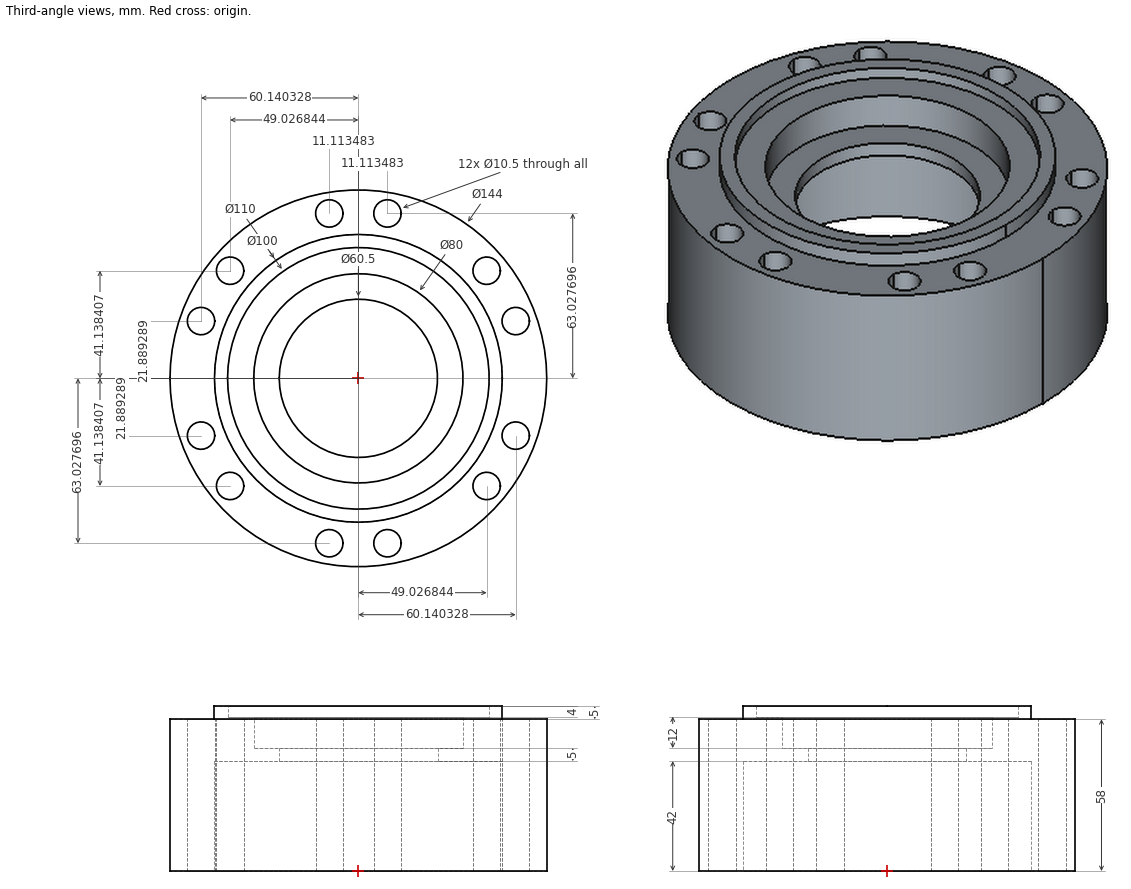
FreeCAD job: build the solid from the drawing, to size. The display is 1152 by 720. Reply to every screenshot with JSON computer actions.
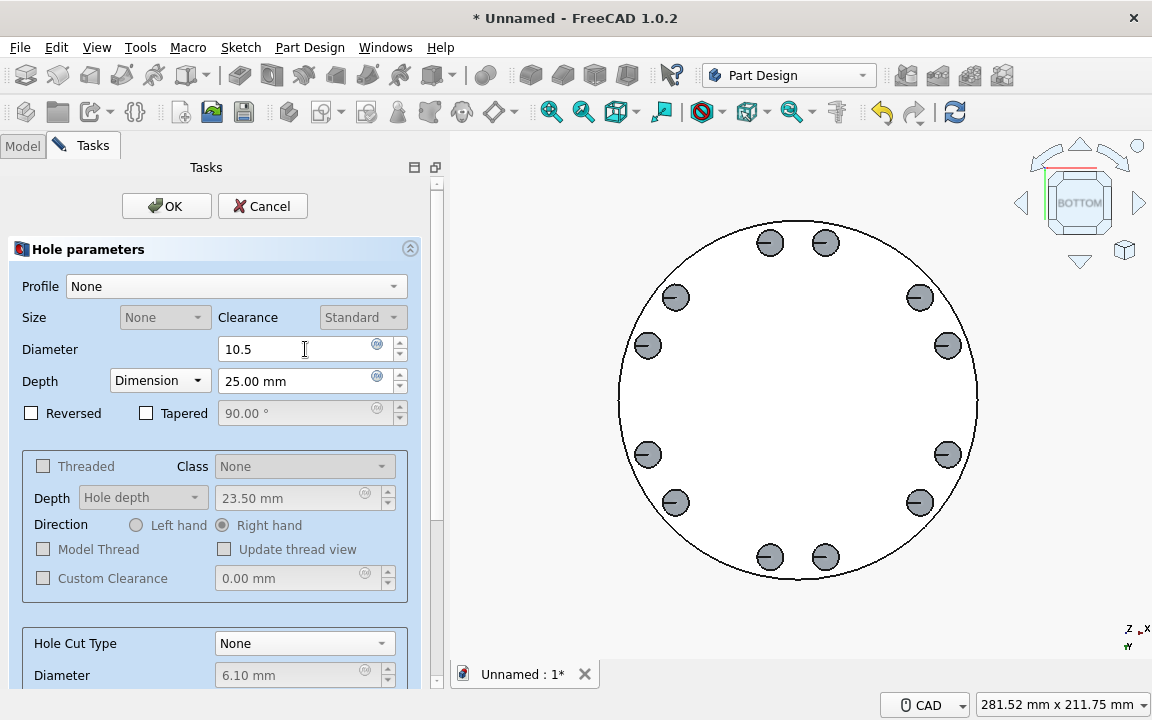
{"action": "left_click", "coordinate": [161, 380]}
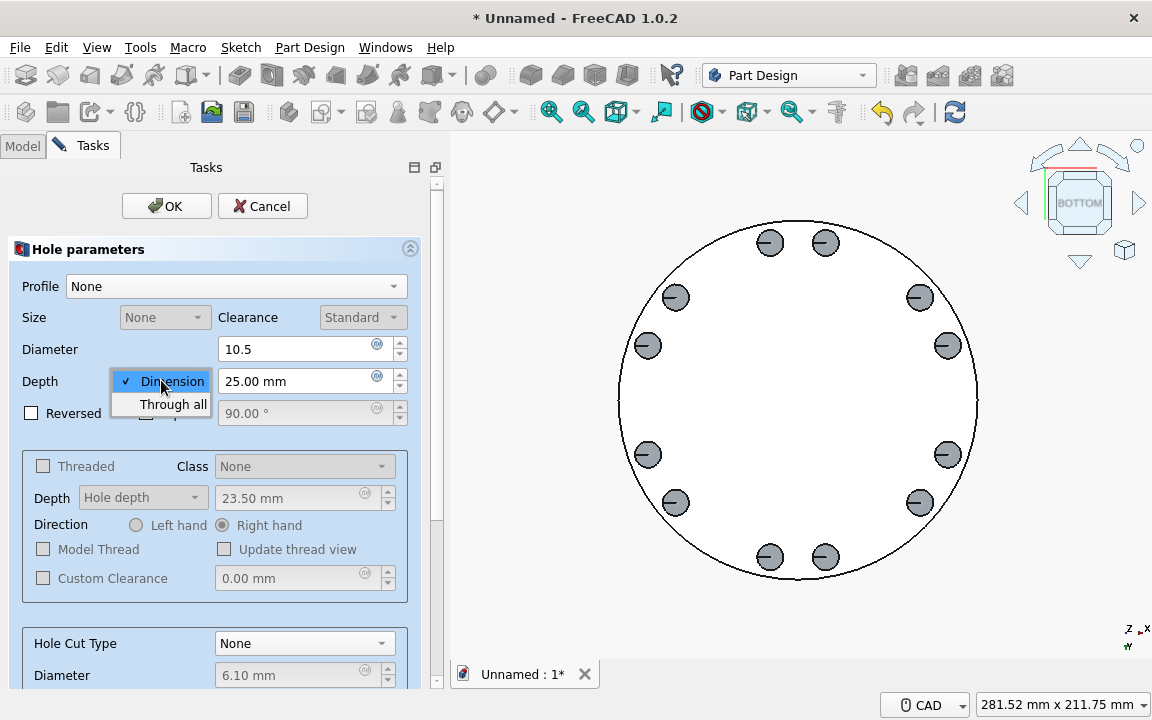
{"action": "left_click", "coordinate": [160, 404]}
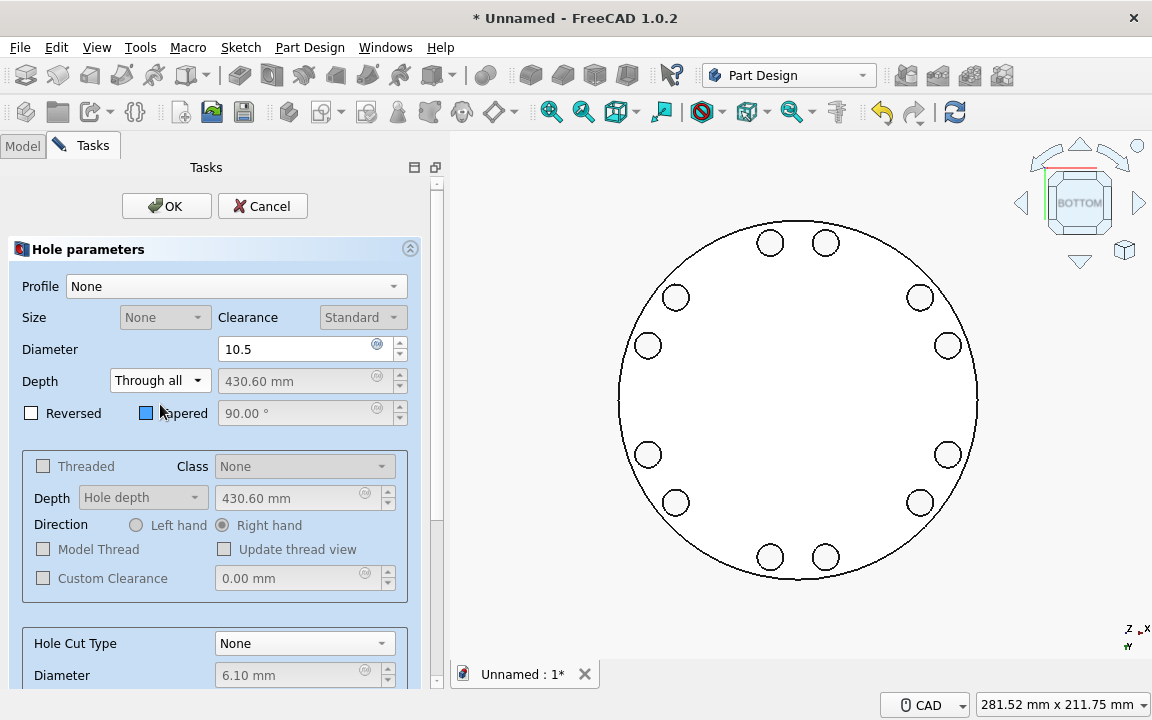
{"action": "left_click", "coordinate": [167, 206]}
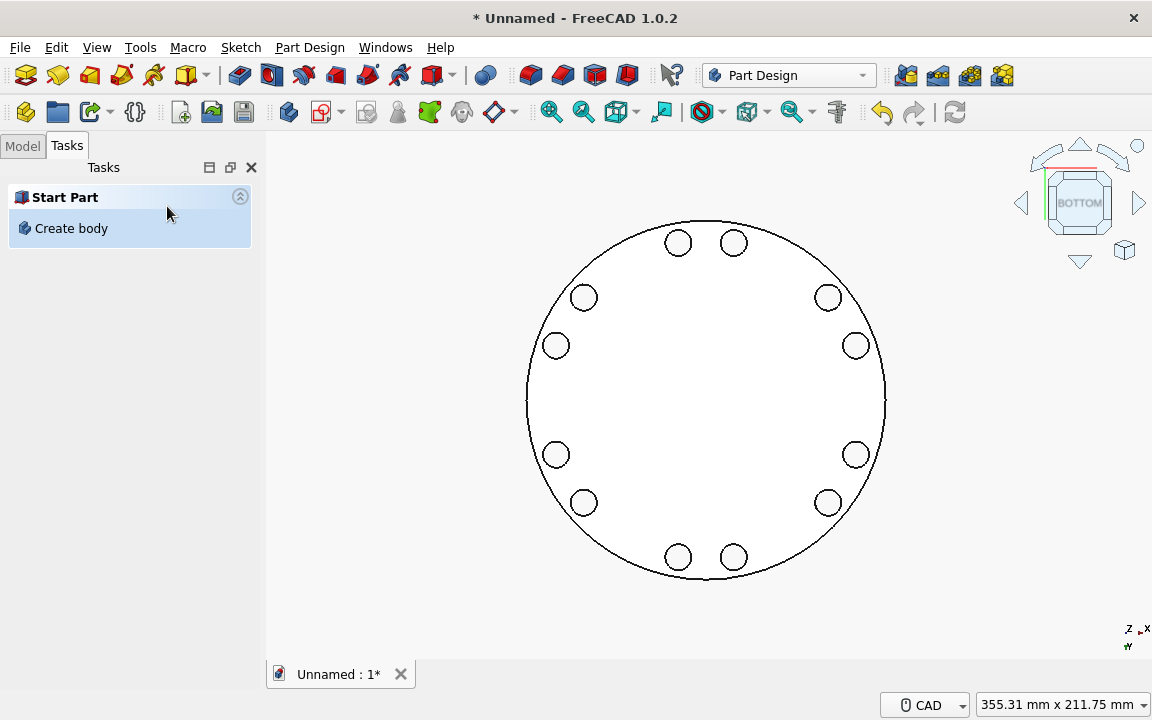
{"action": "left_click", "coordinate": [706, 399]}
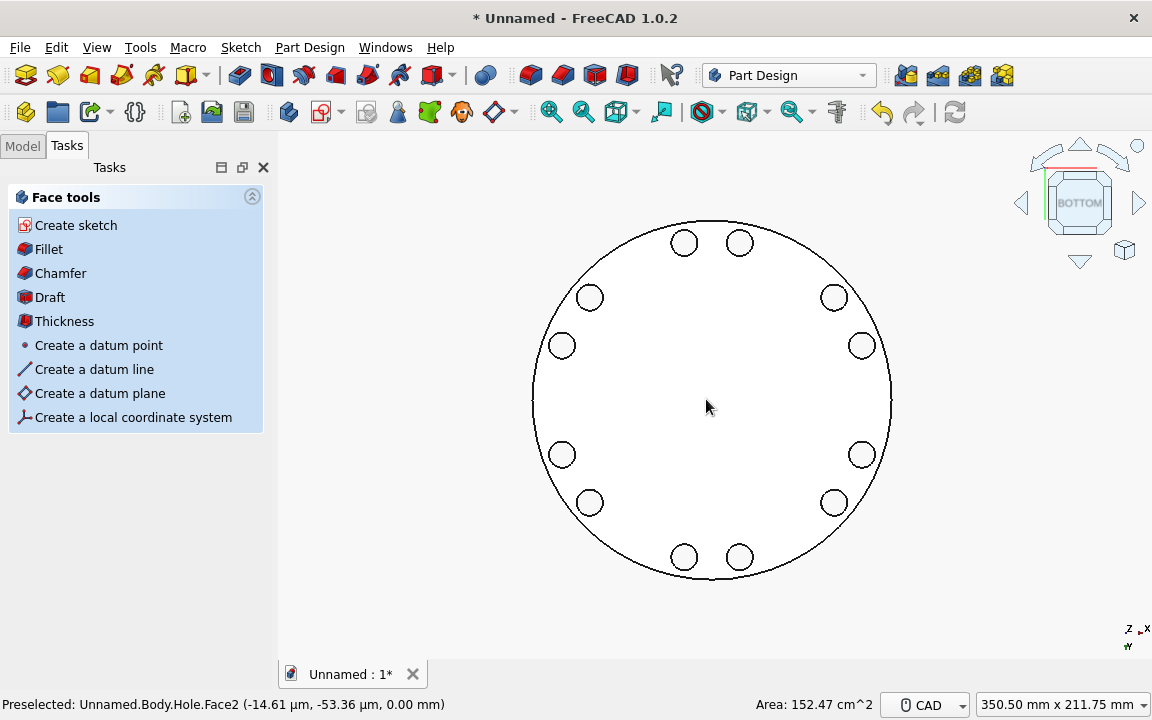
{"action": "left_click", "coordinate": [322, 112]}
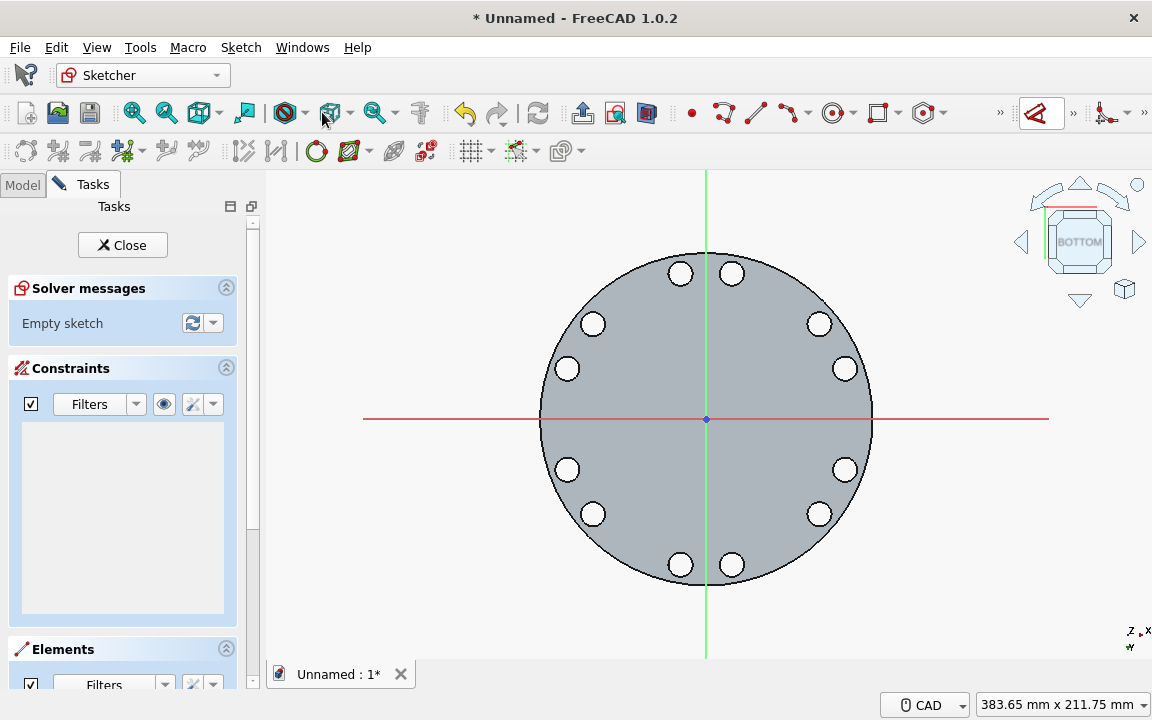
{"action": "key", "text": "g c"}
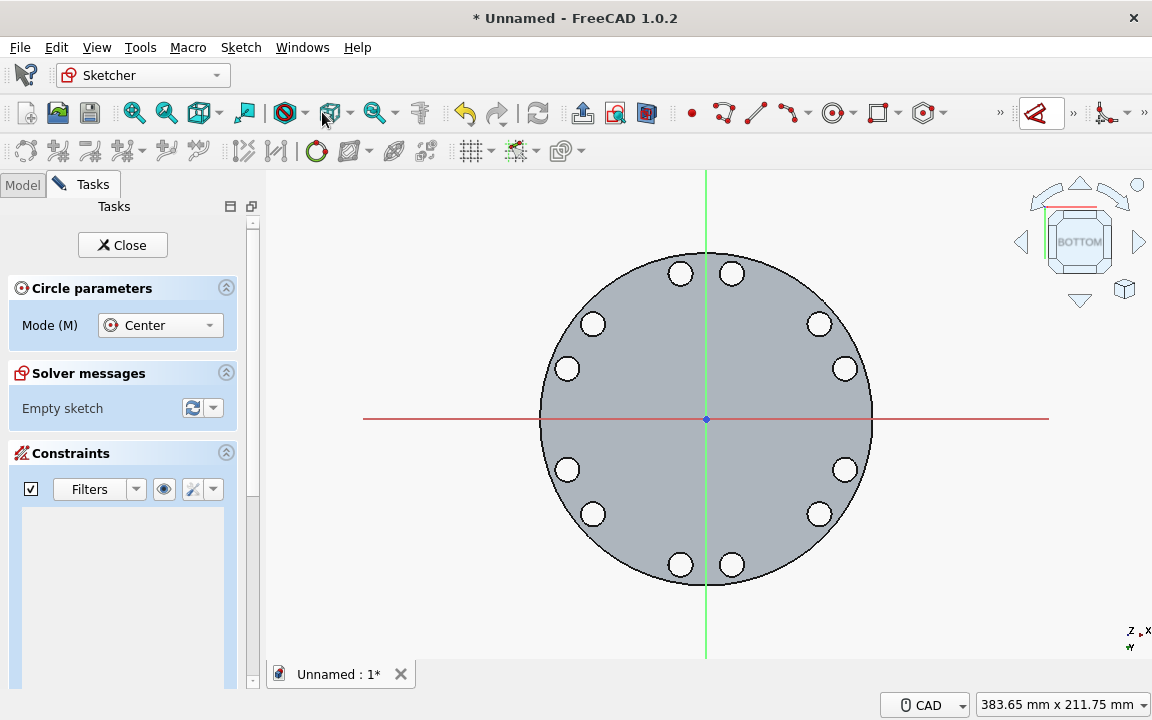
{"action": "left_click", "coordinate": [706, 419]}
{"action": "left_click", "coordinate": [796, 329]}
{"action": "key", "text": "Escape"}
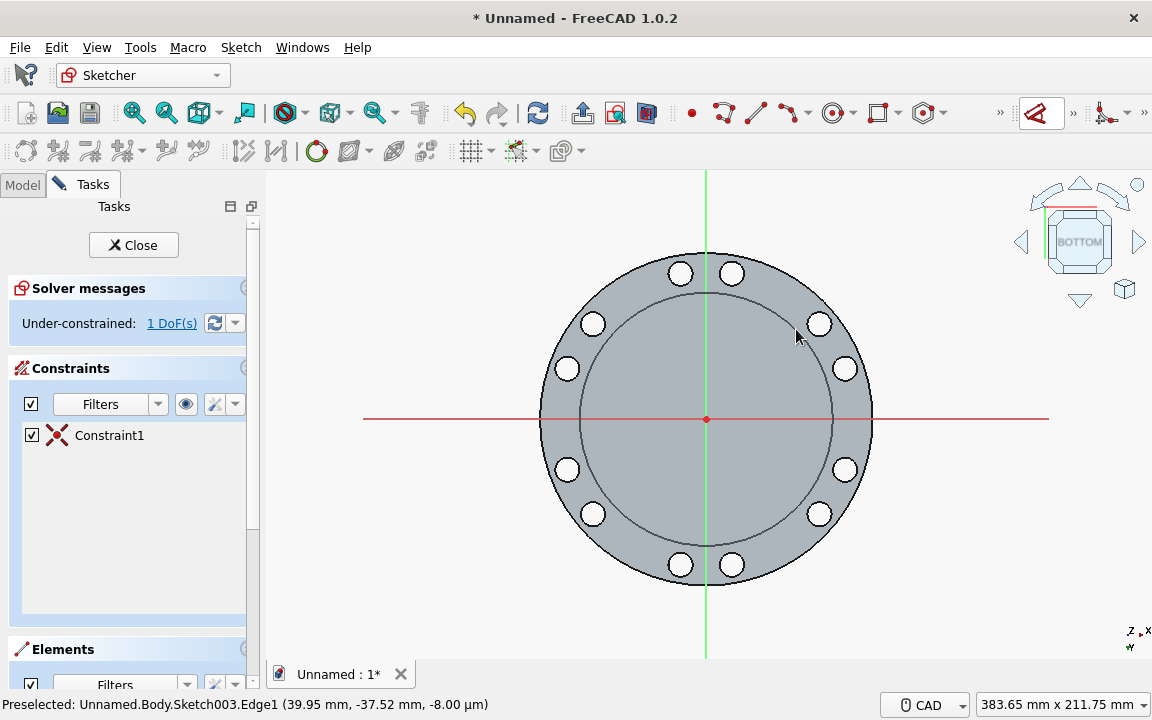
{"action": "key", "text": "d"}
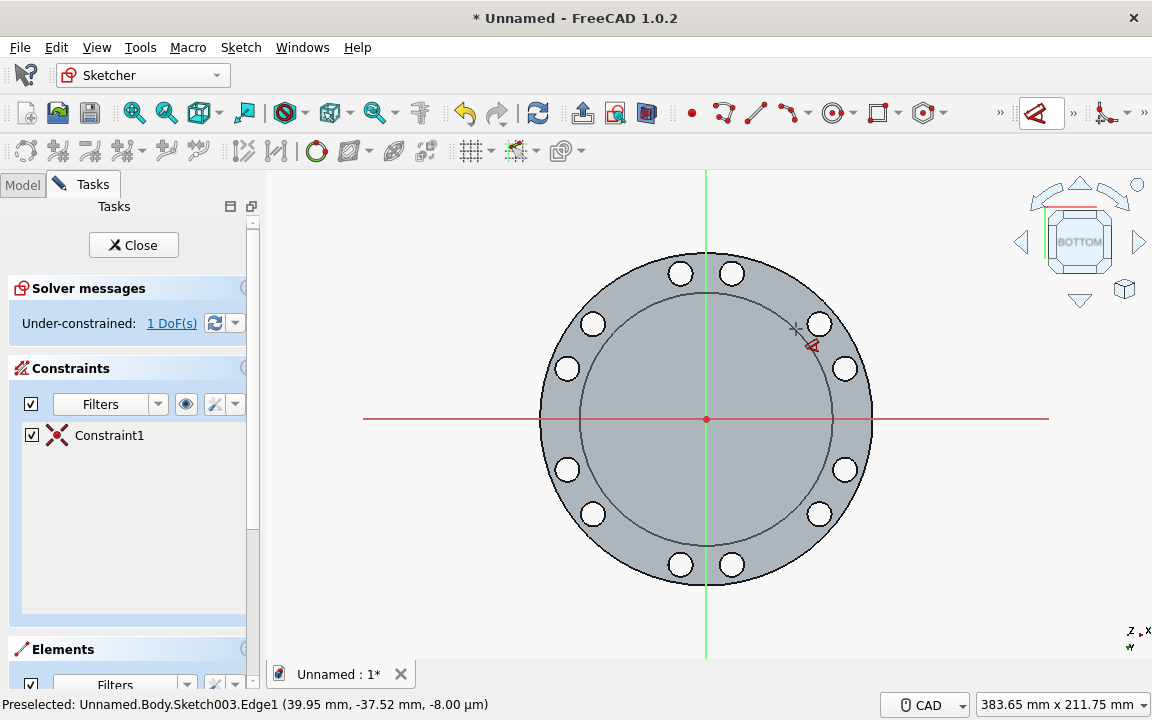
{"action": "left_click", "coordinate": [795, 329]}
{"action": "left_click", "coordinate": [817, 306]}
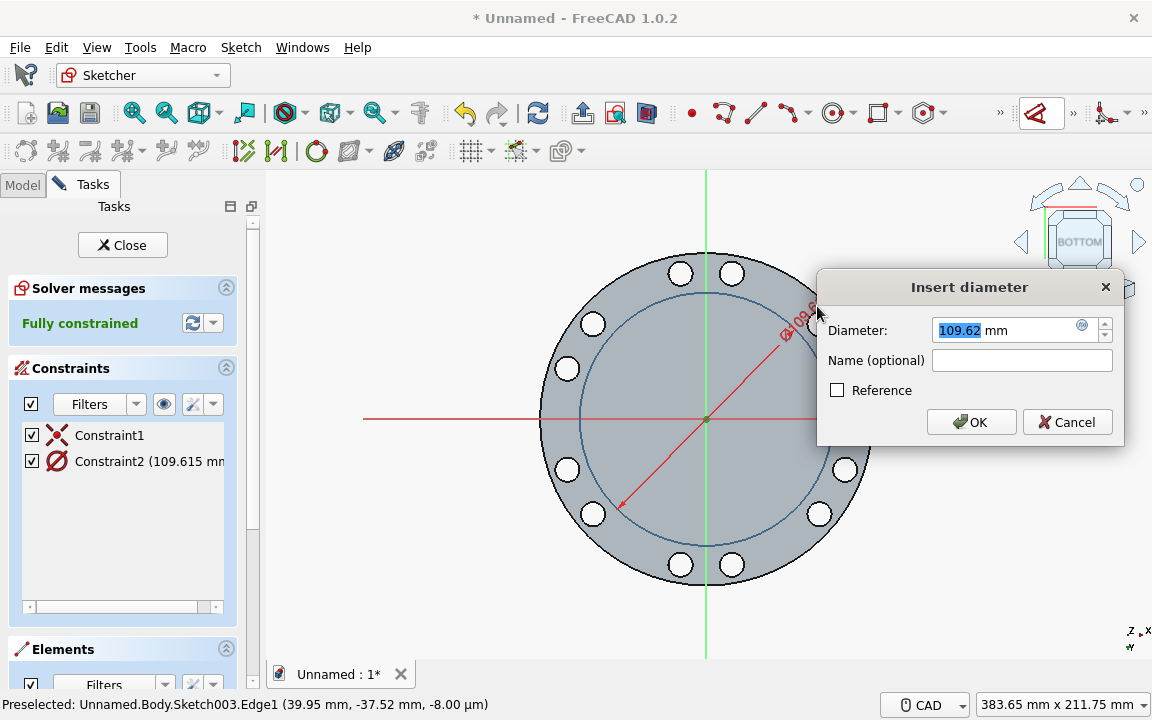
{"action": "type", "text": "110"}
{"action": "key", "text": "Return"}
{"action": "key", "text": "Escape"}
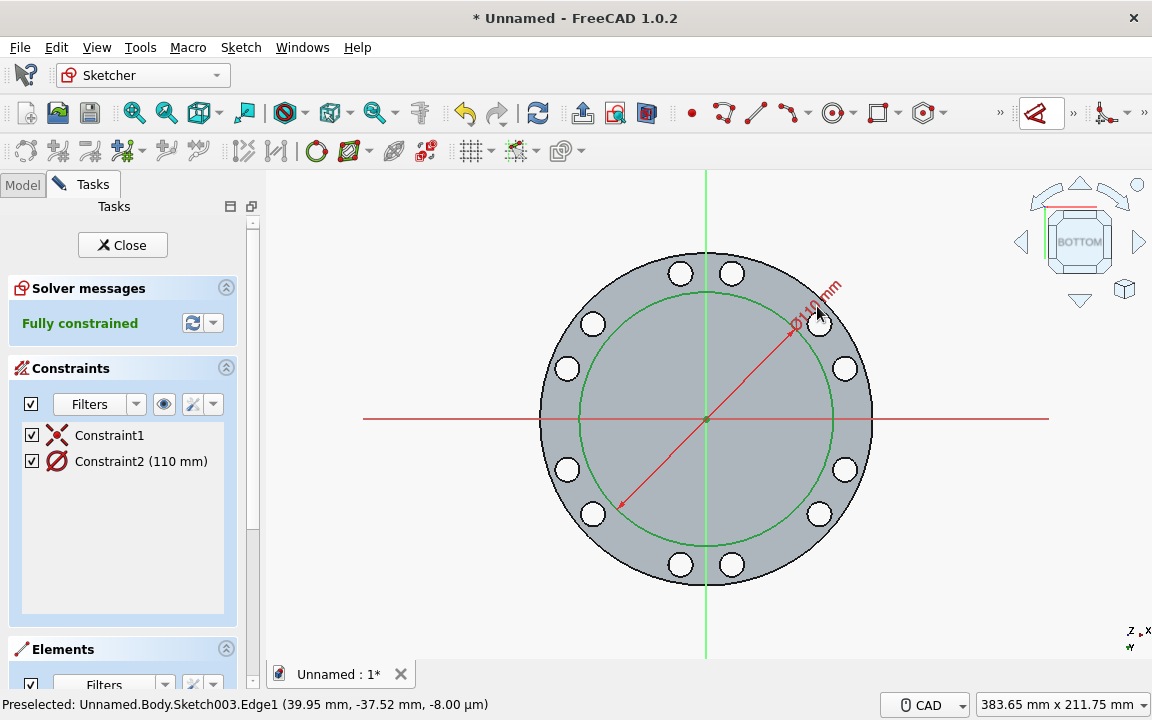
{"action": "left_click", "coordinate": [123, 245]}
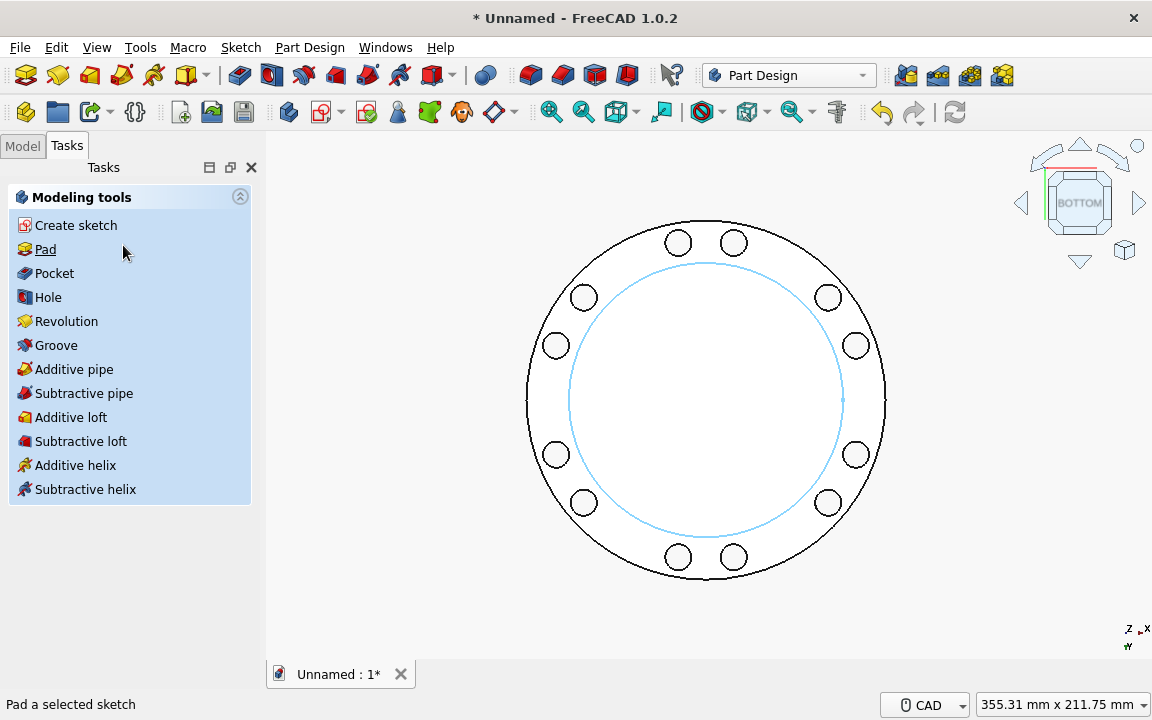
{"action": "left_click", "coordinate": [240, 76]}